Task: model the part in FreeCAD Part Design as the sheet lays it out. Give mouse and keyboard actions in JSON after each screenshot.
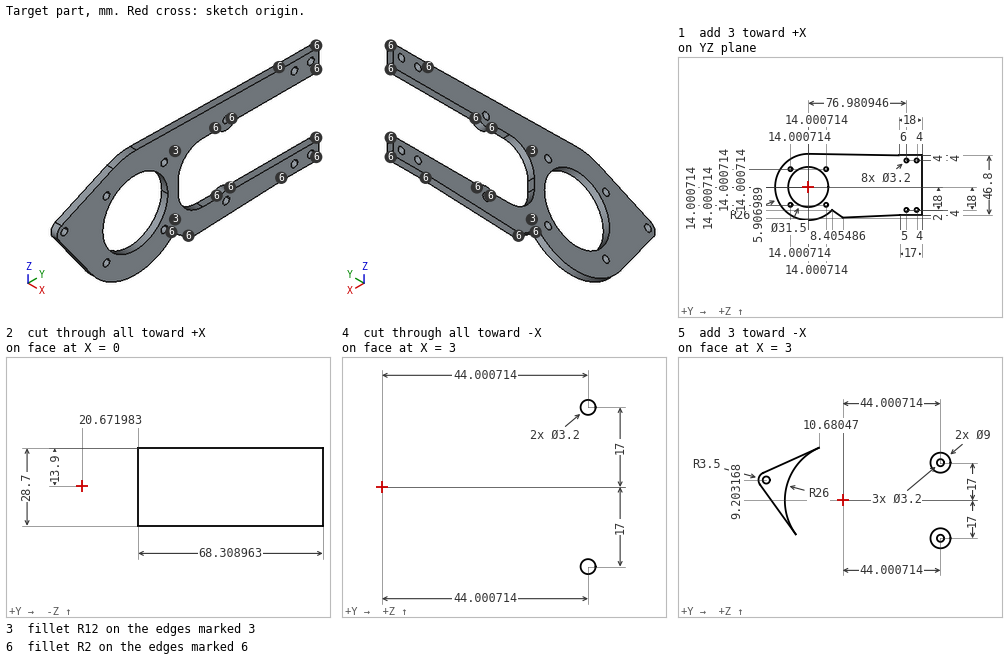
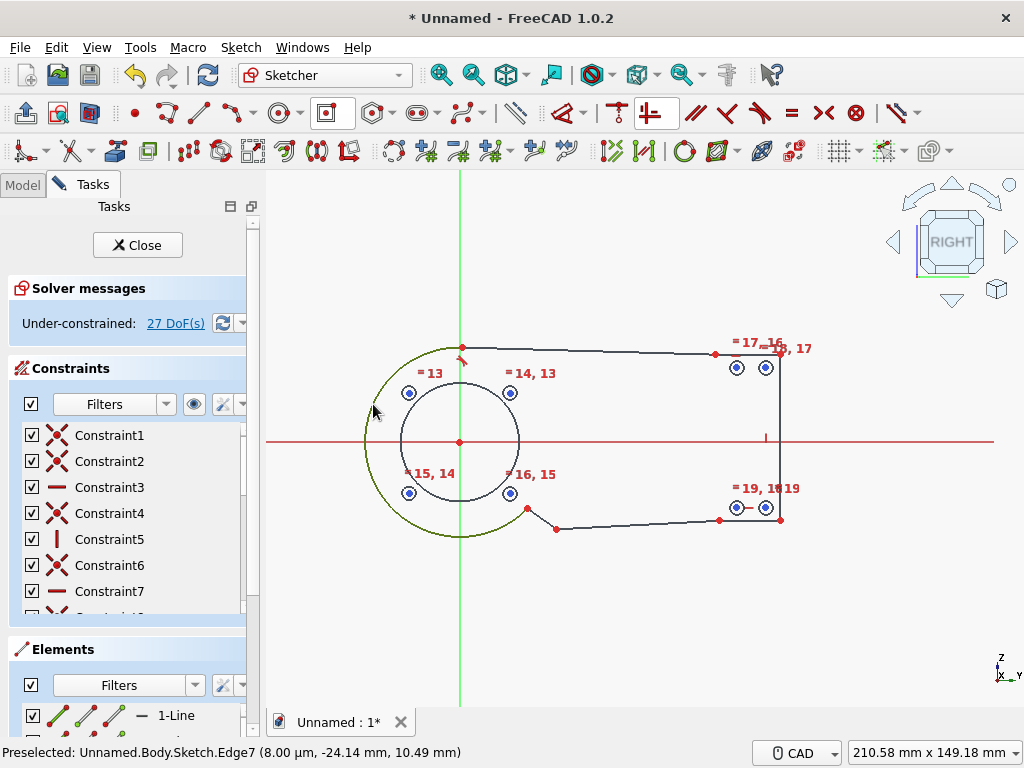
{"action": "left_click", "coordinate": [586, 114]}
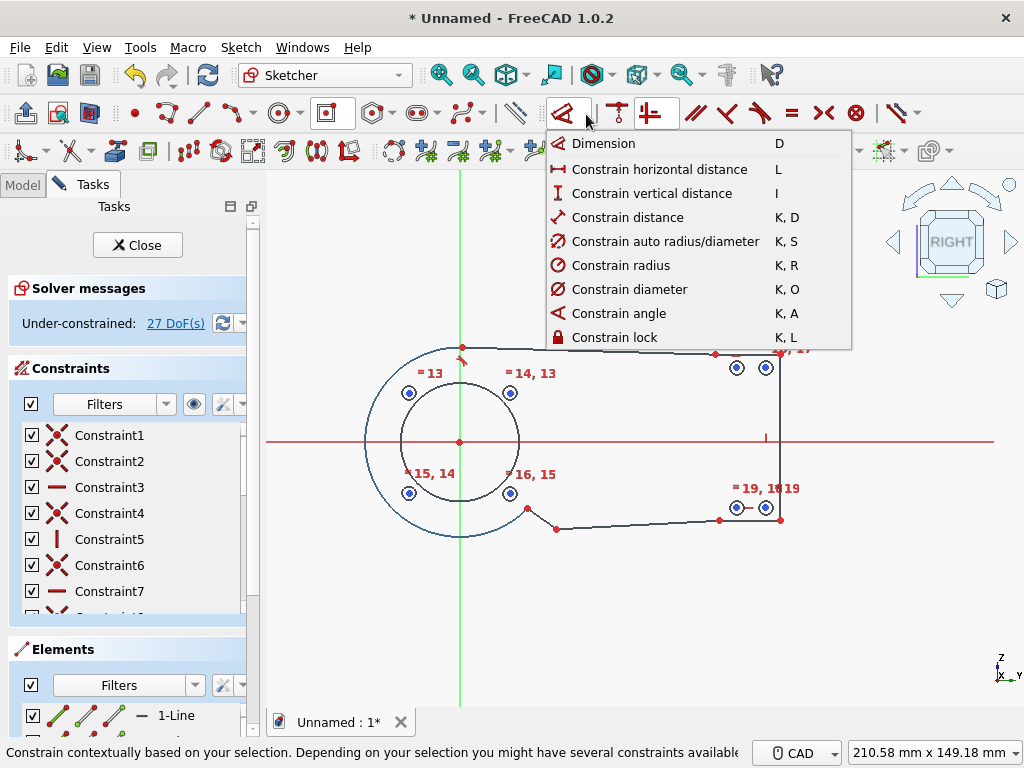
{"action": "left_click", "coordinate": [699, 265]}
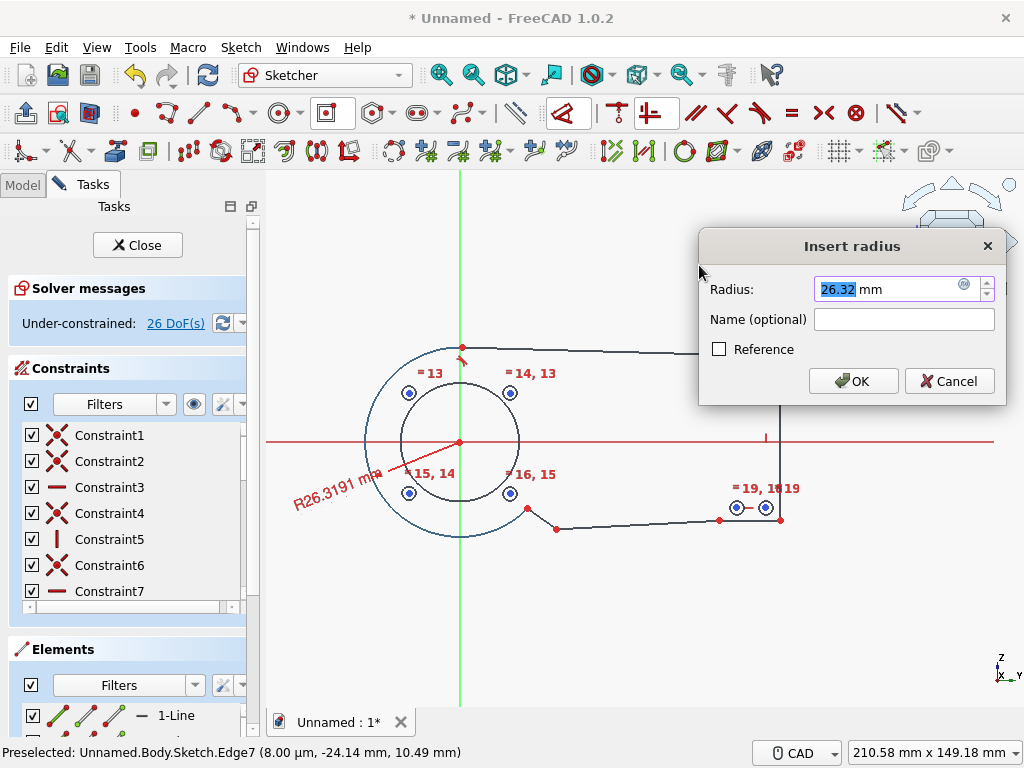
{"action": "type", "text": "26"}
{"action": "key", "text": "Return"}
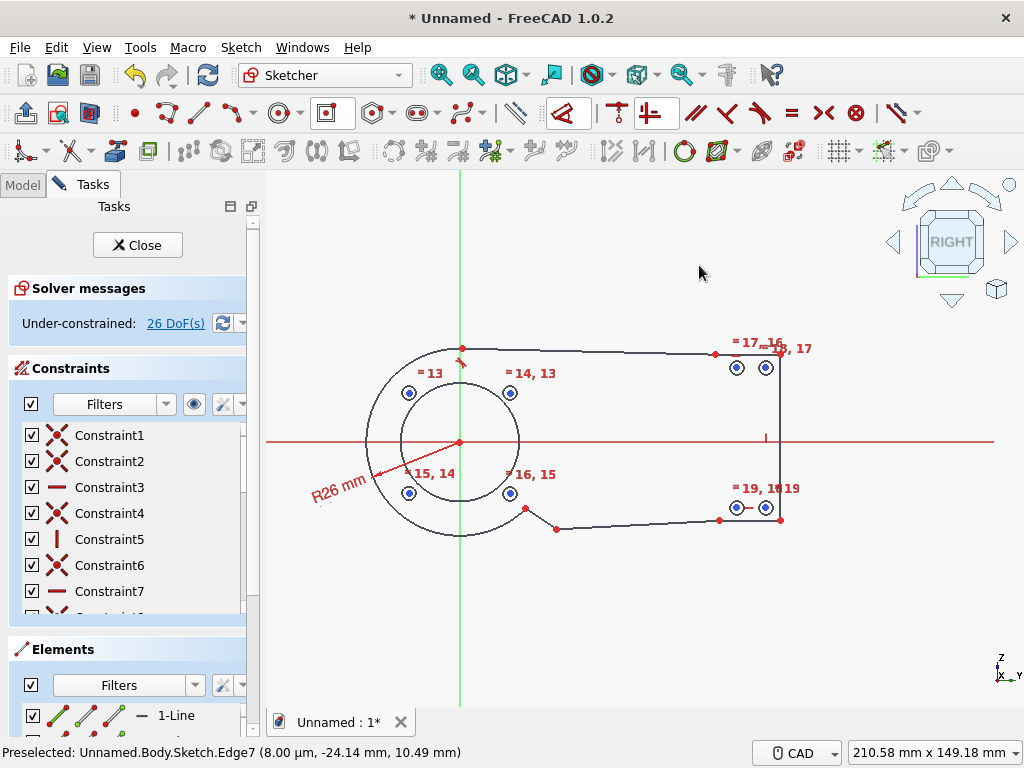
{"action": "scroll", "coordinate": [404, 388], "scroll_direction": "up", "scroll_amount": 7}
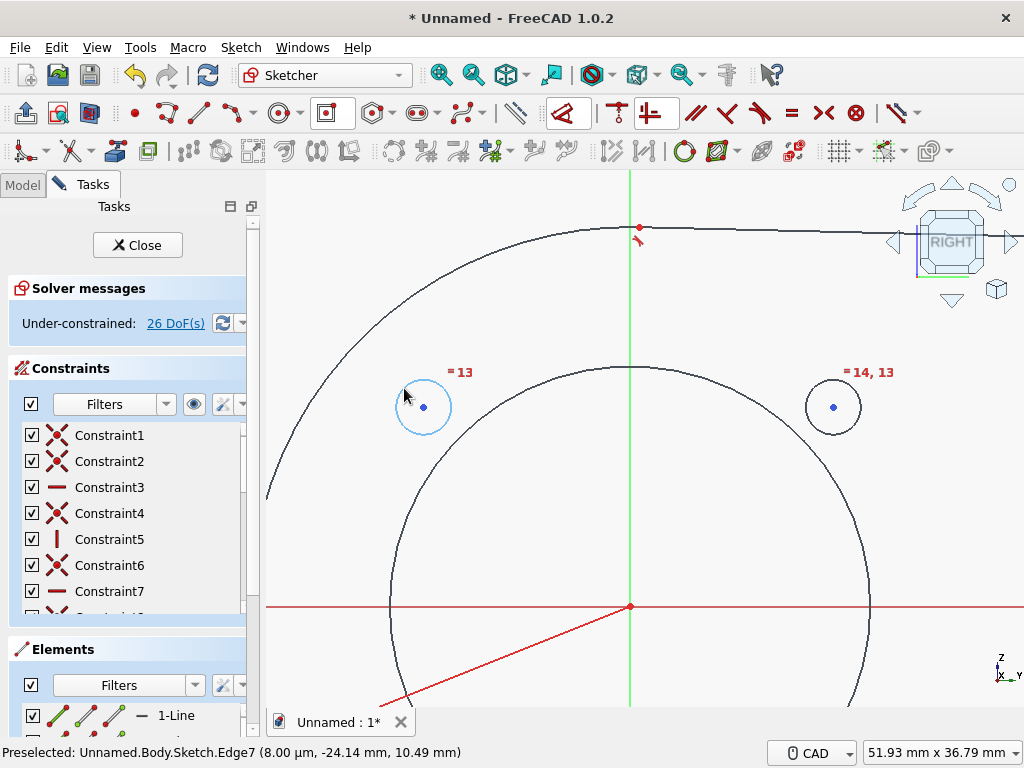
{"action": "left_click", "coordinate": [404, 388]}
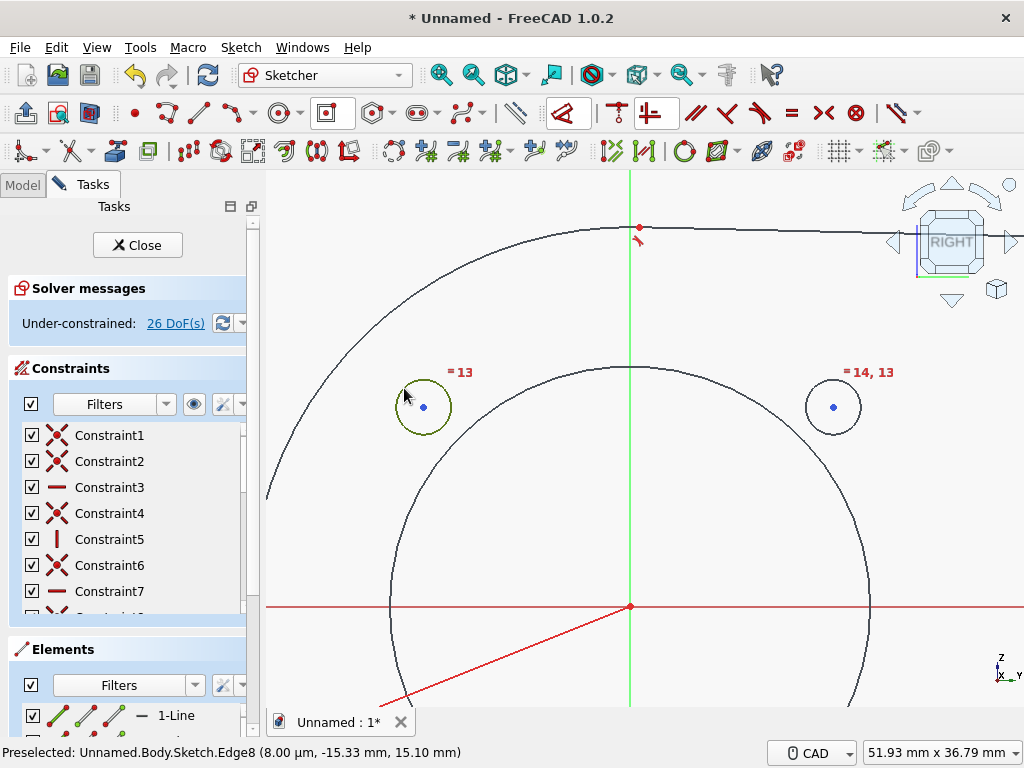
{"action": "left_click", "coordinate": [586, 114]}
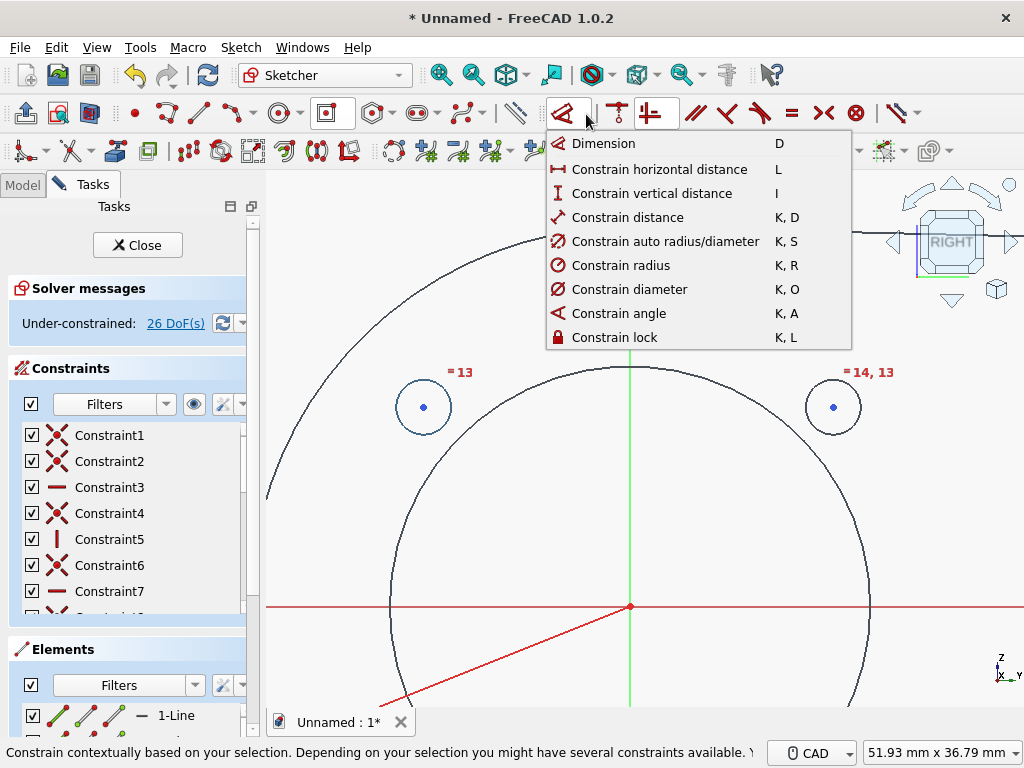
{"action": "left_click", "coordinate": [699, 289]}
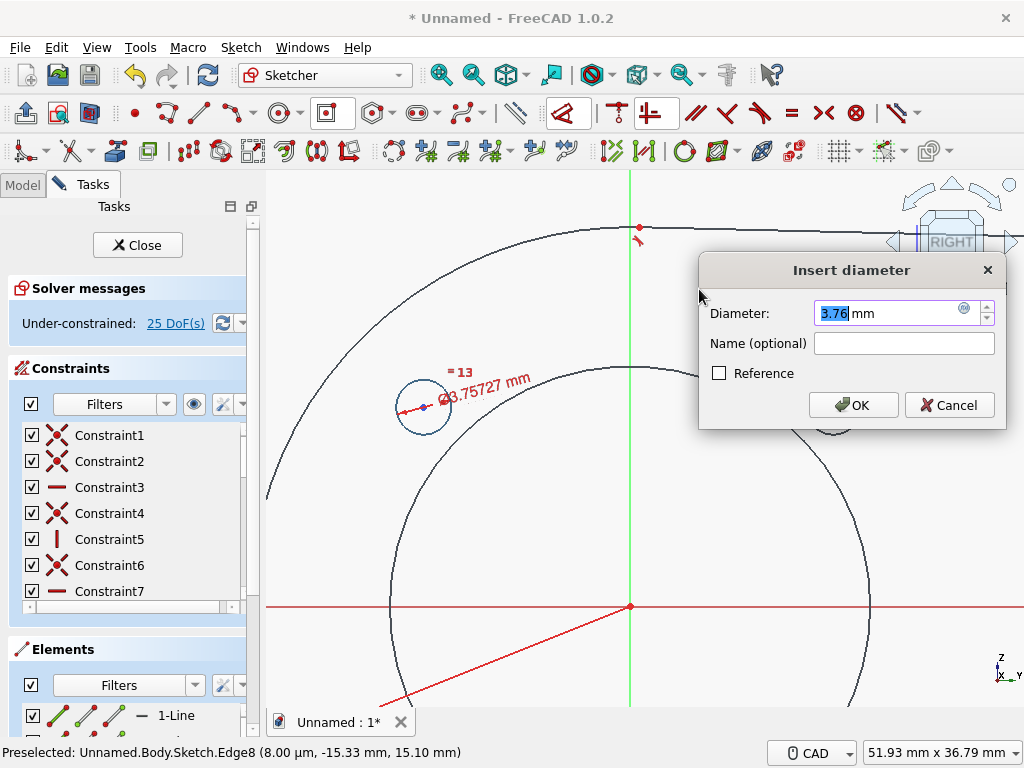
{"action": "type", "text": "3.2"}
{"action": "key", "text": "Return"}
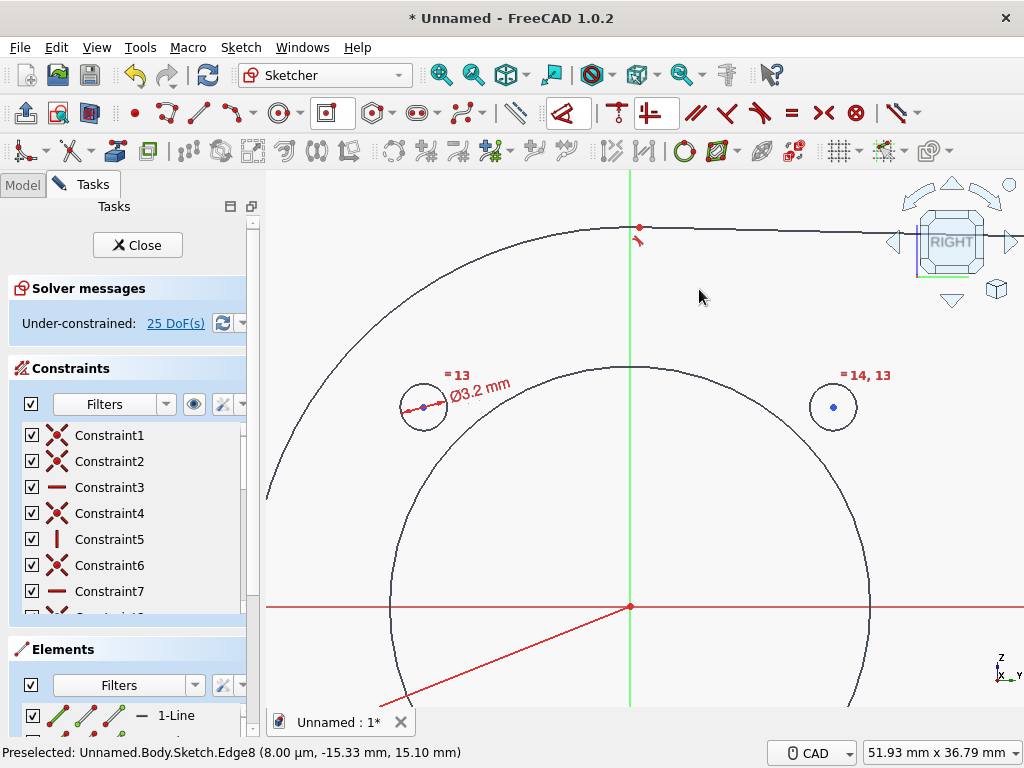
{"action": "left_click", "coordinate": [799, 436]}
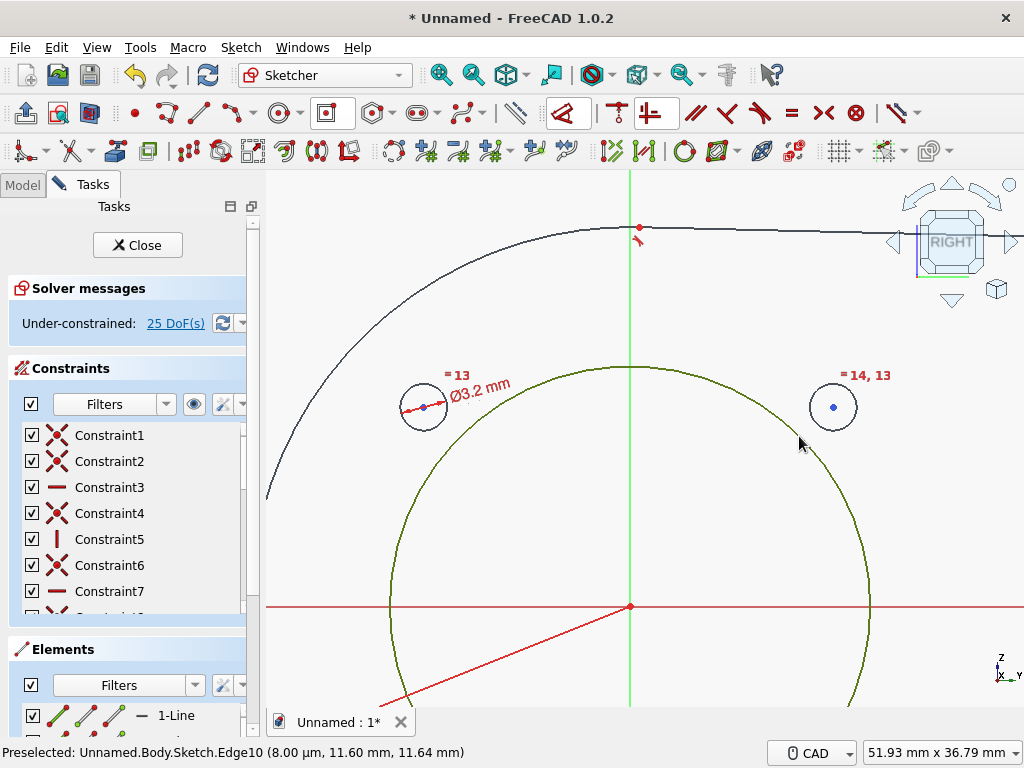
{"action": "left_click", "coordinate": [586, 114]}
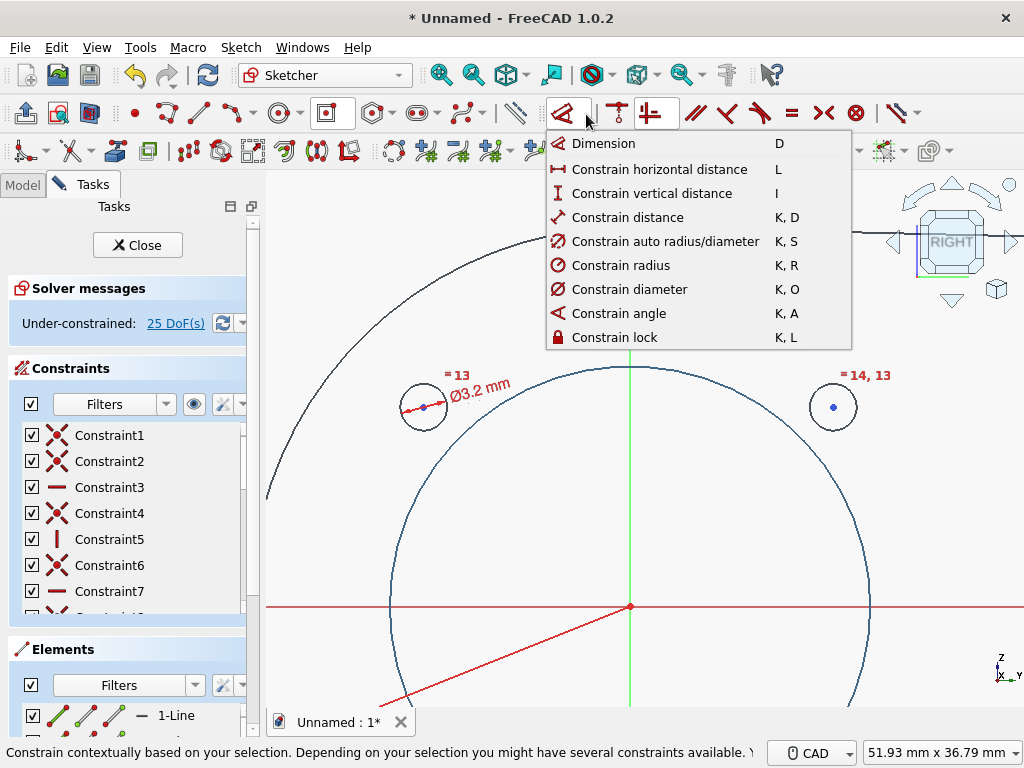
{"action": "left_click", "coordinate": [699, 289]}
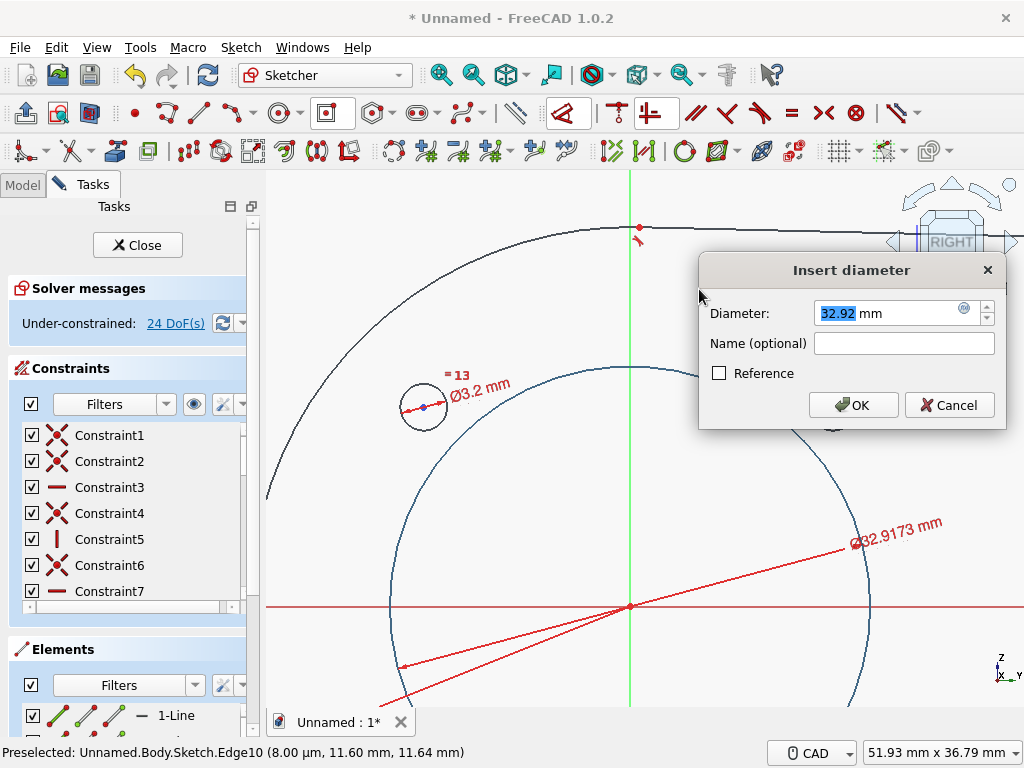
{"action": "type", "text": "31.5"}
{"action": "key", "text": "Return"}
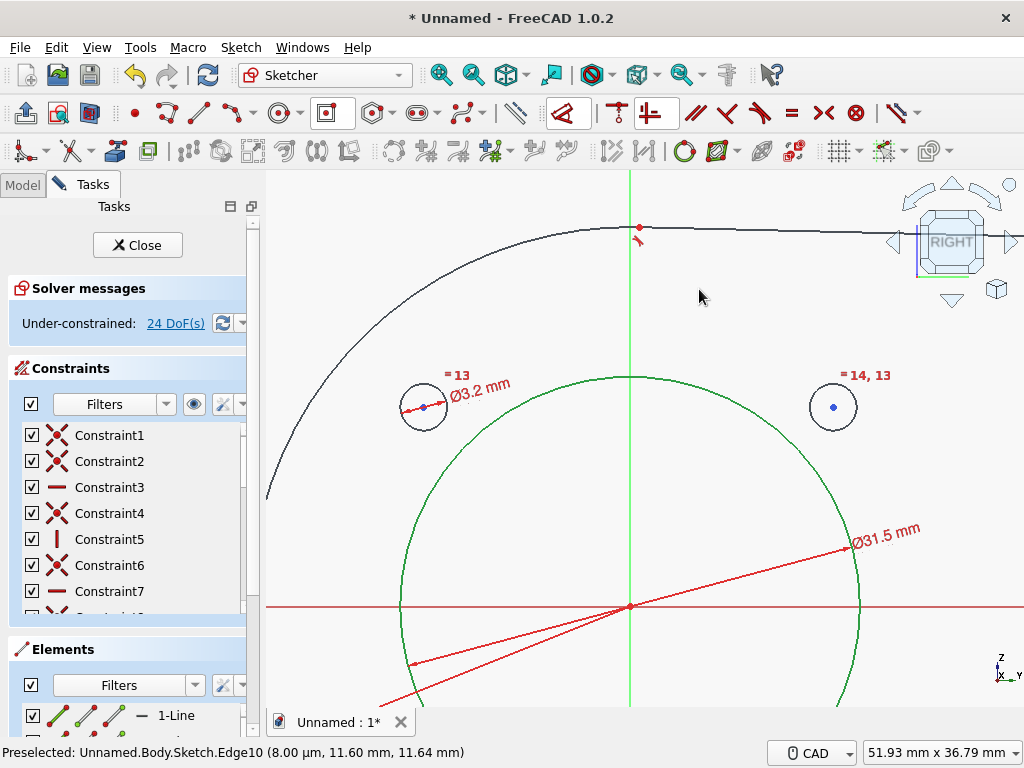
{"action": "scroll", "coordinate": [404, 388], "scroll_direction": "down", "scroll_amount": 7}